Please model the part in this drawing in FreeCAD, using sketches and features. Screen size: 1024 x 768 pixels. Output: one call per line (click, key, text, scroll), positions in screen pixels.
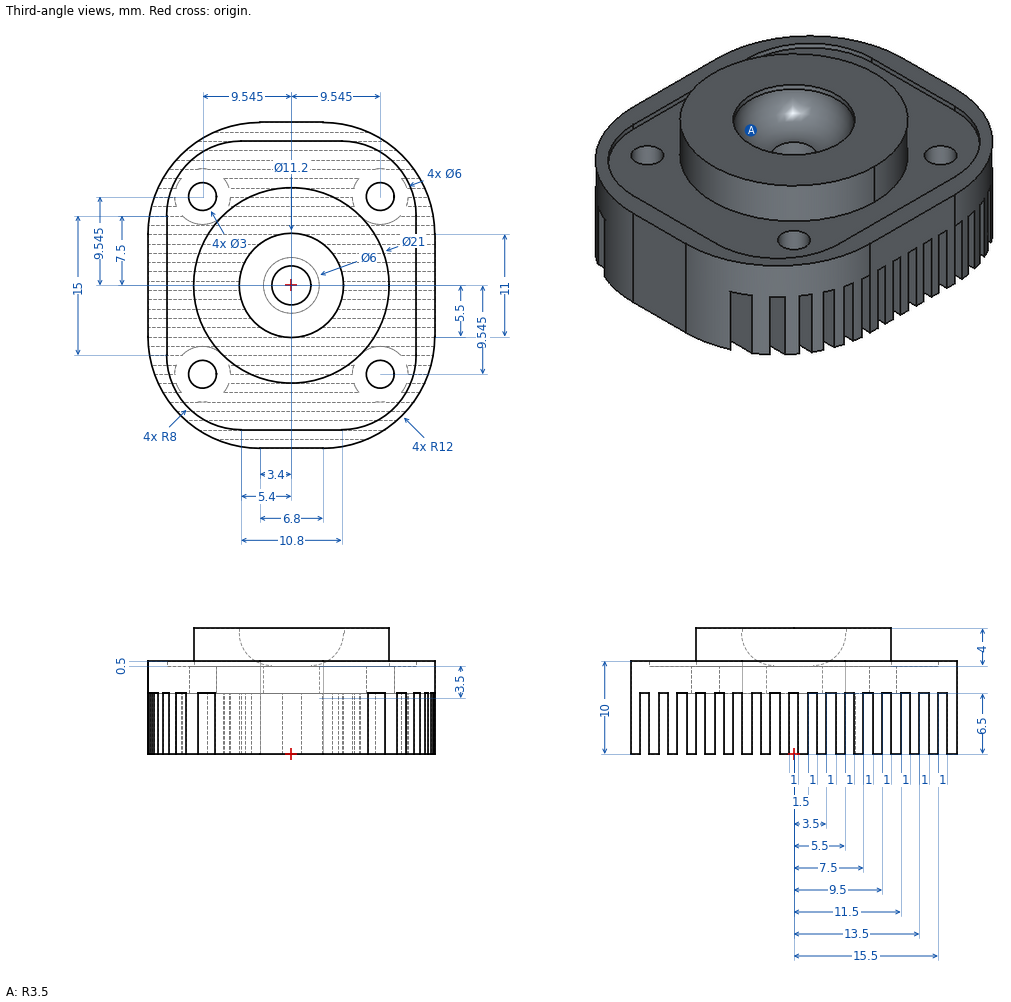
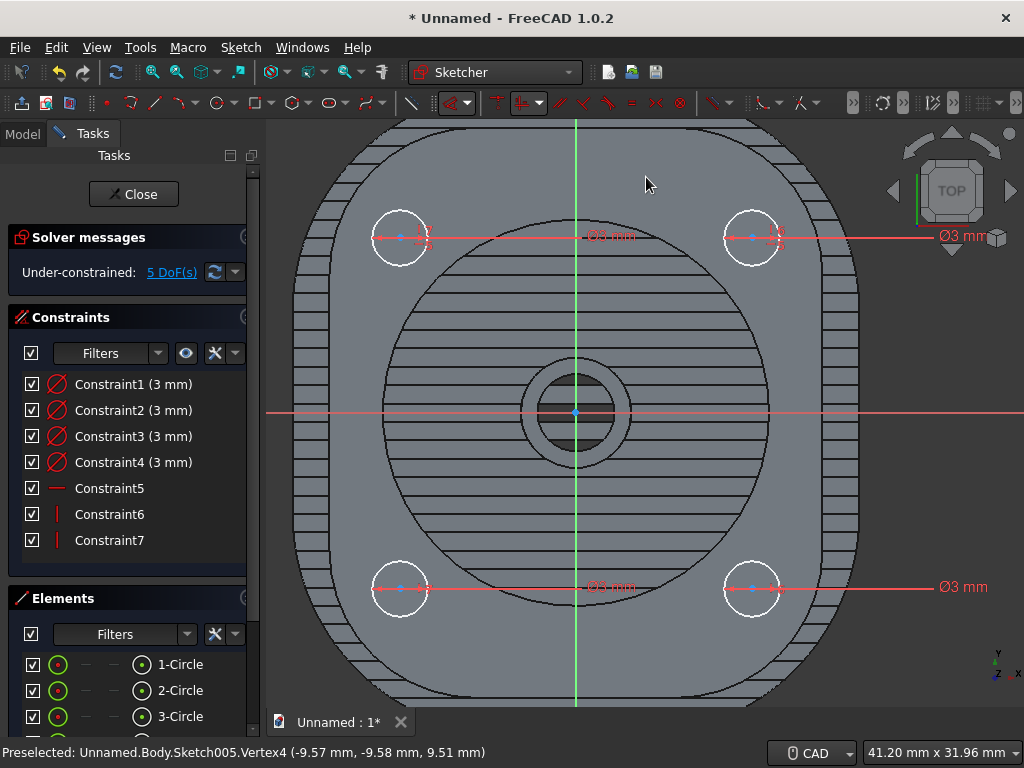
click(752, 589)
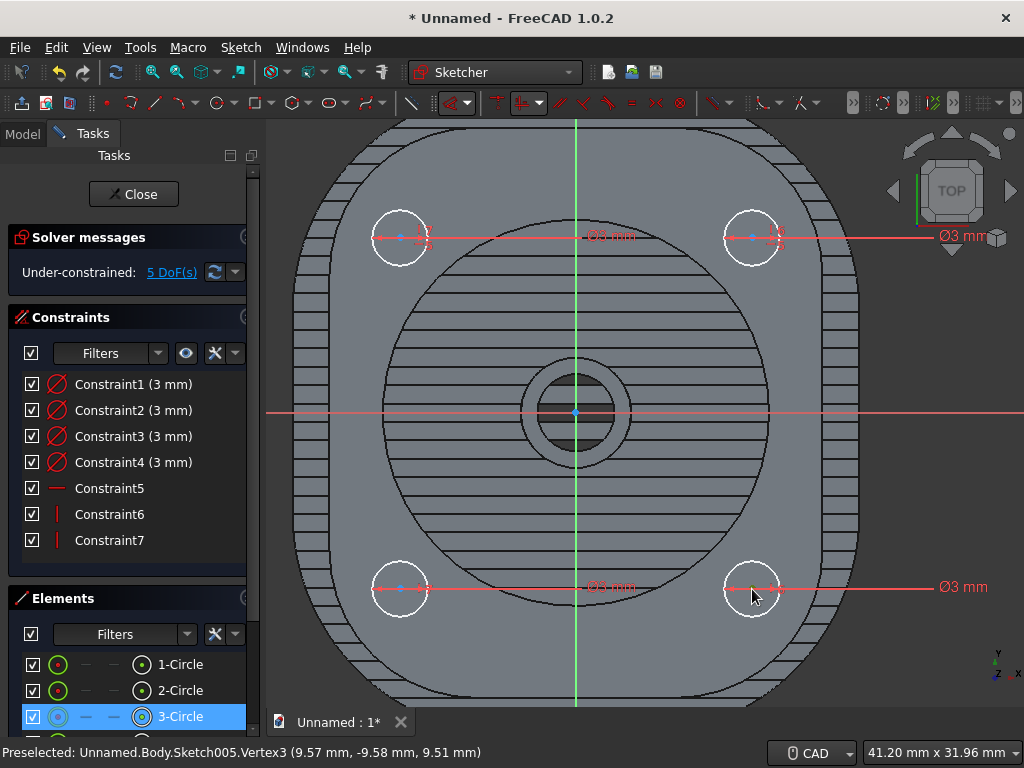
click(400, 589)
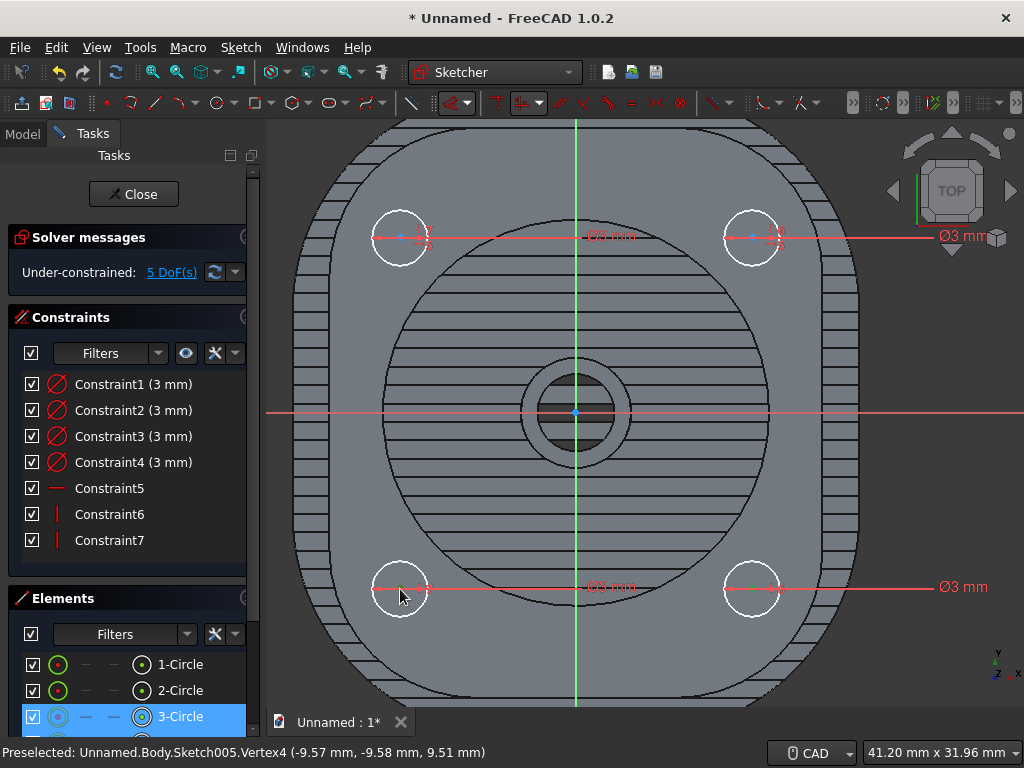
click(542, 104)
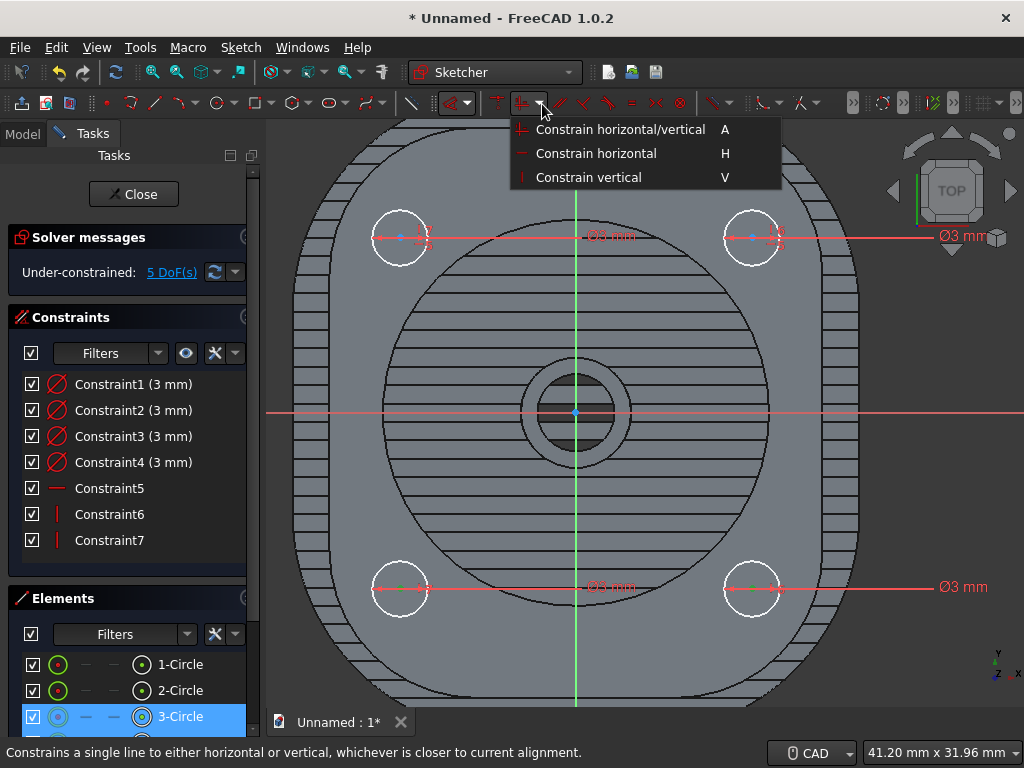
click(646, 153)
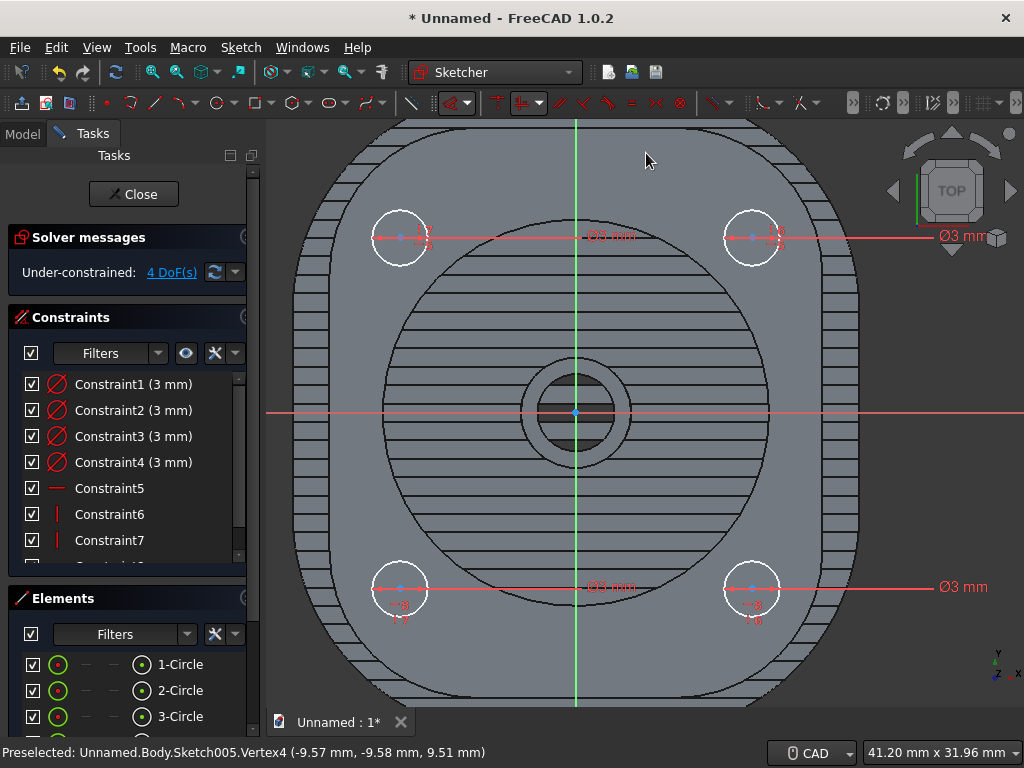
click(400, 238)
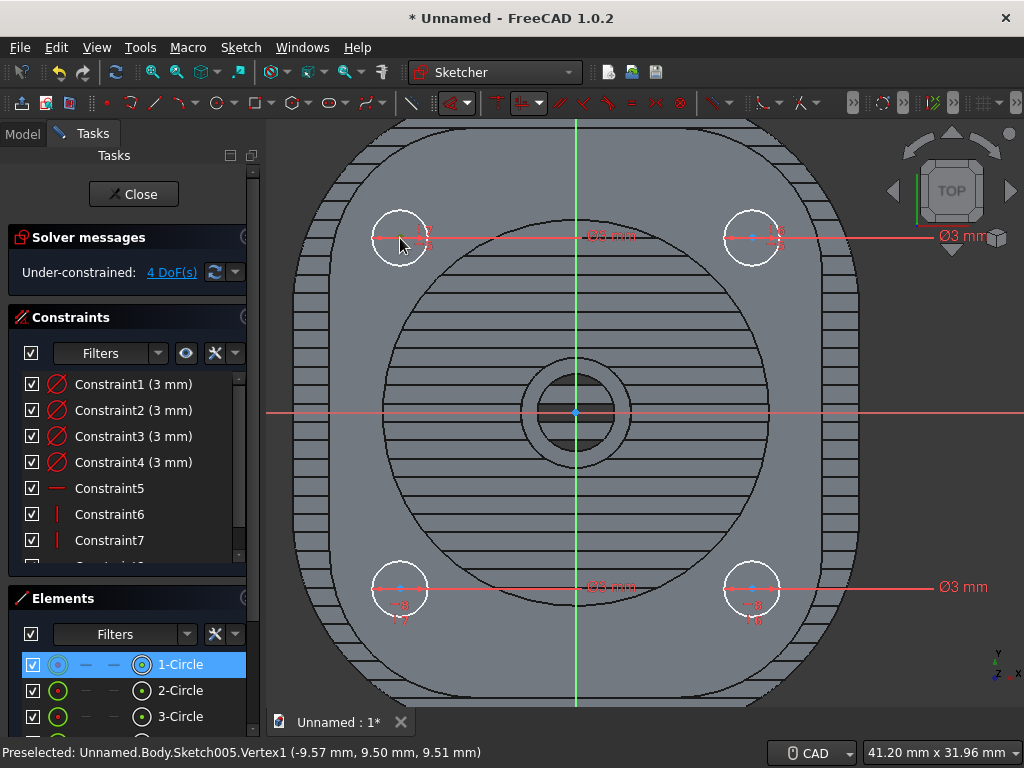
key(l)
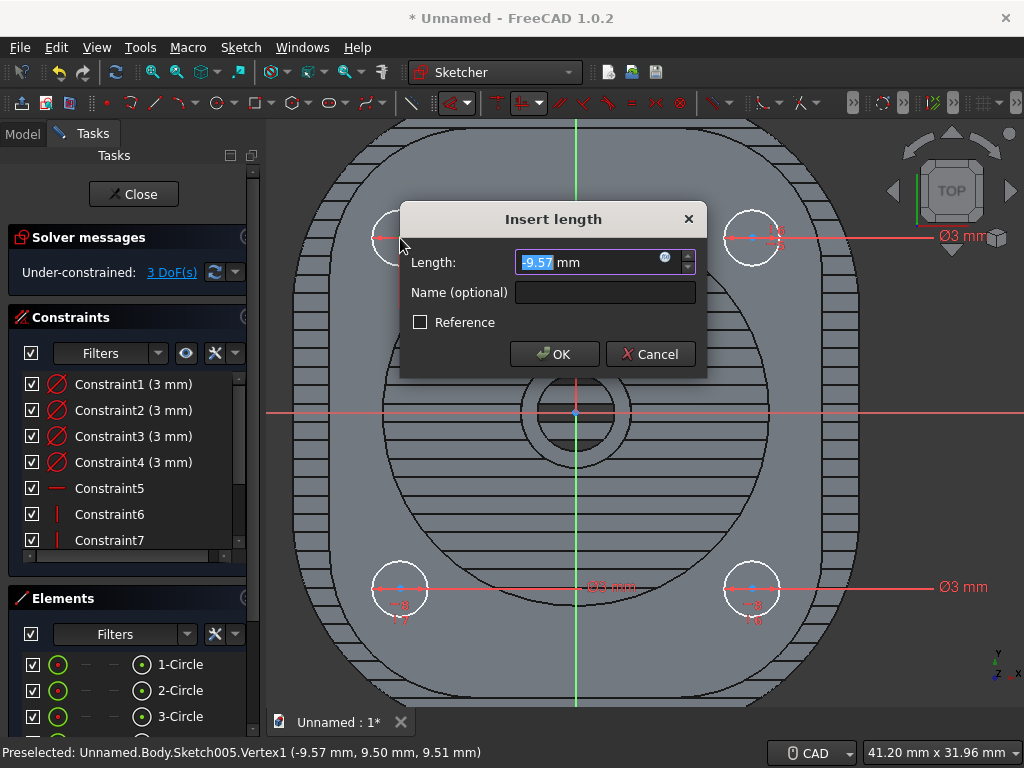
text(-9.545)
key(Return)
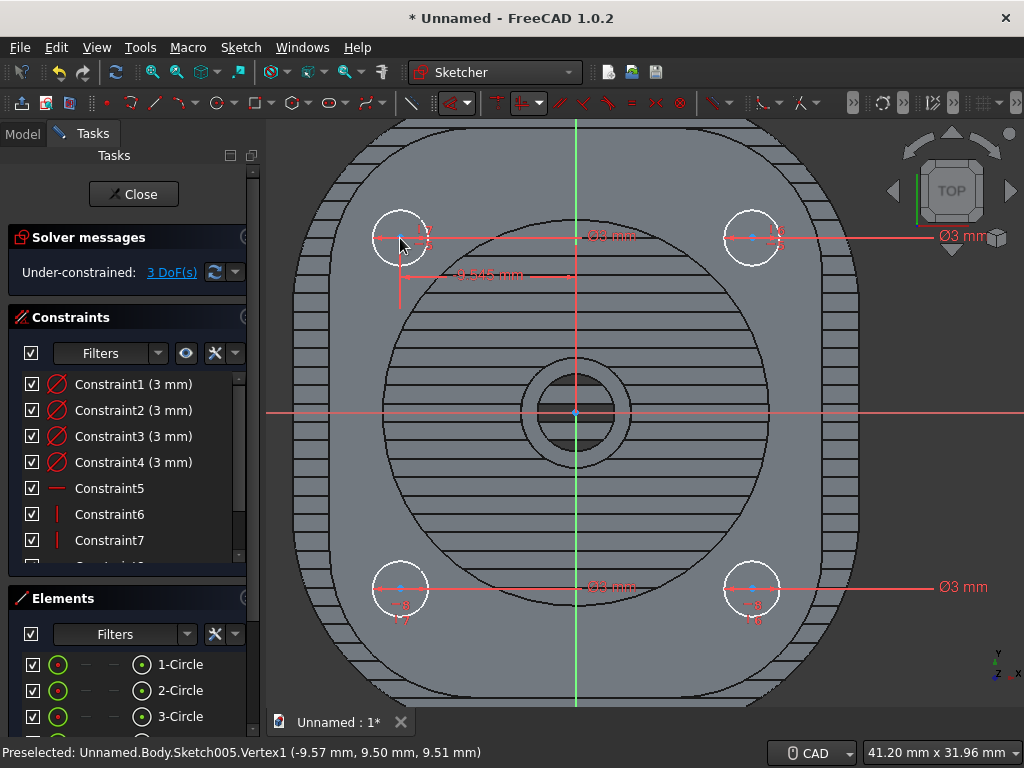
click(400, 238)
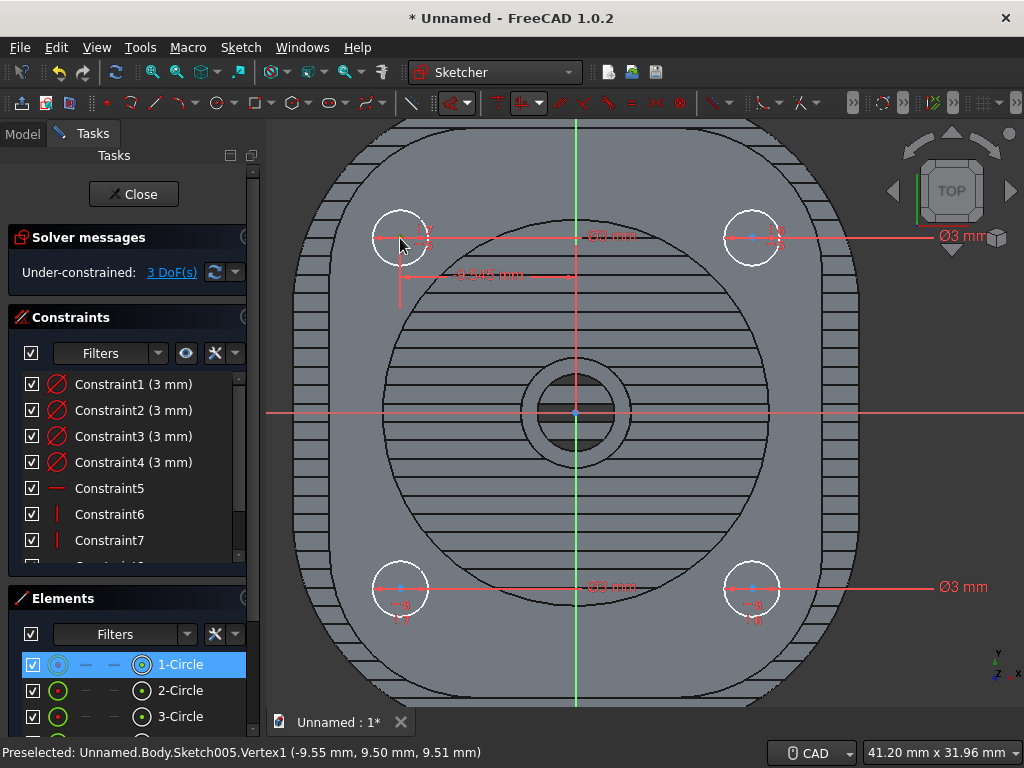
key(i)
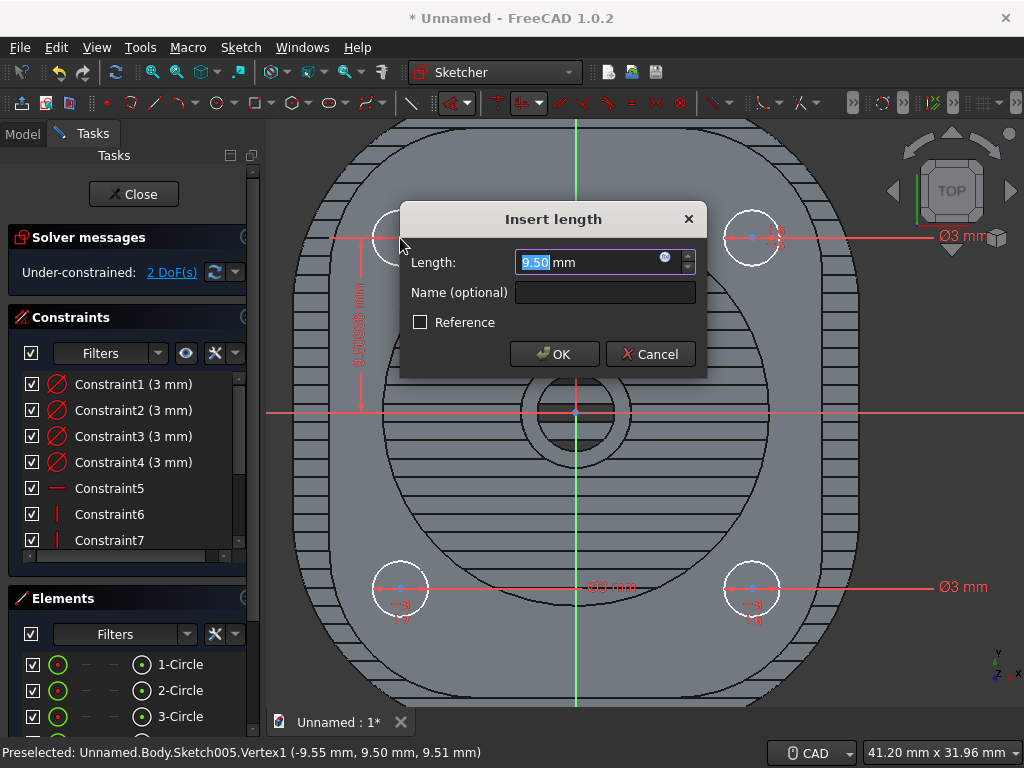
text(9.545)
key(Return)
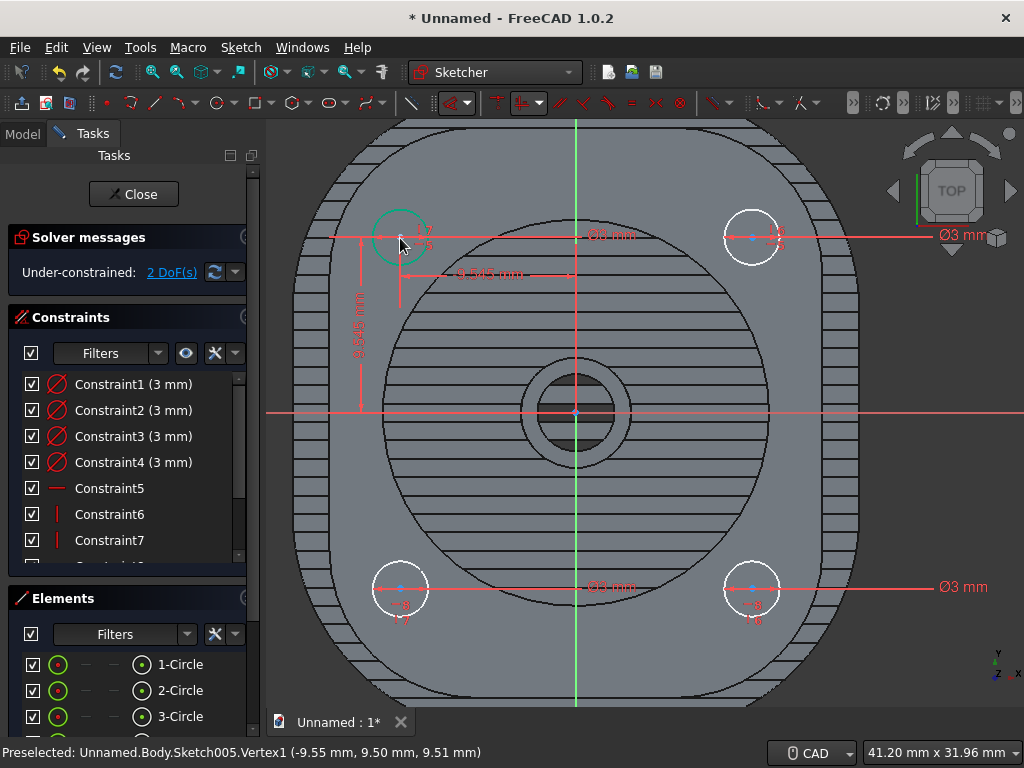
click(752, 237)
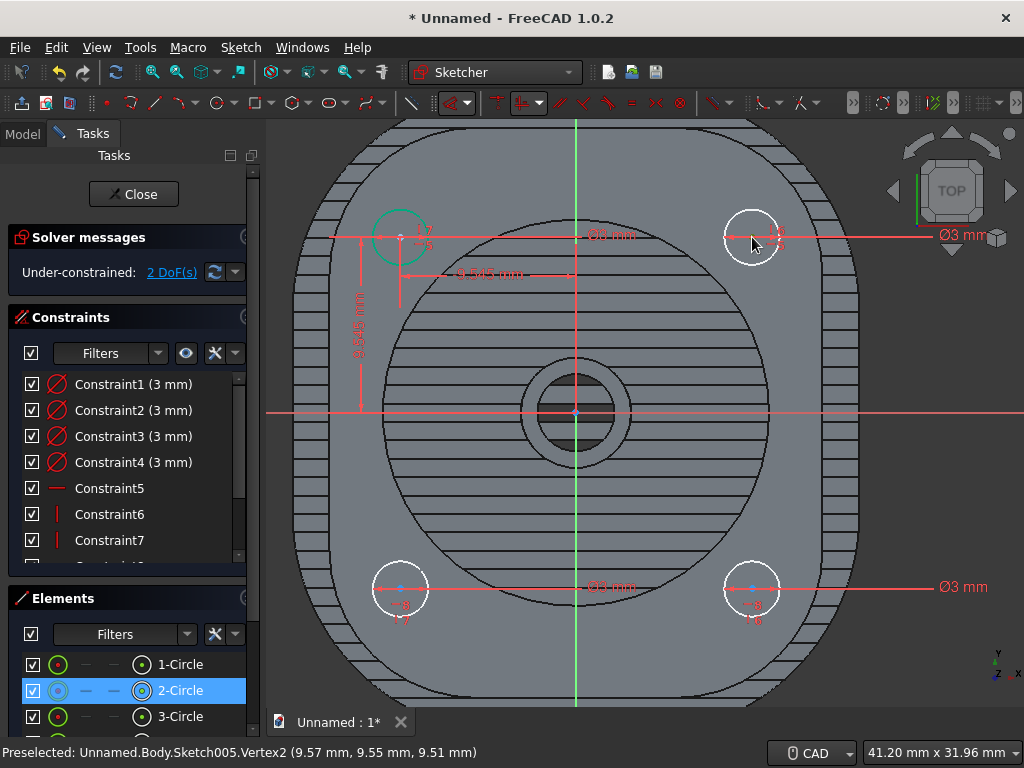
click(470, 104)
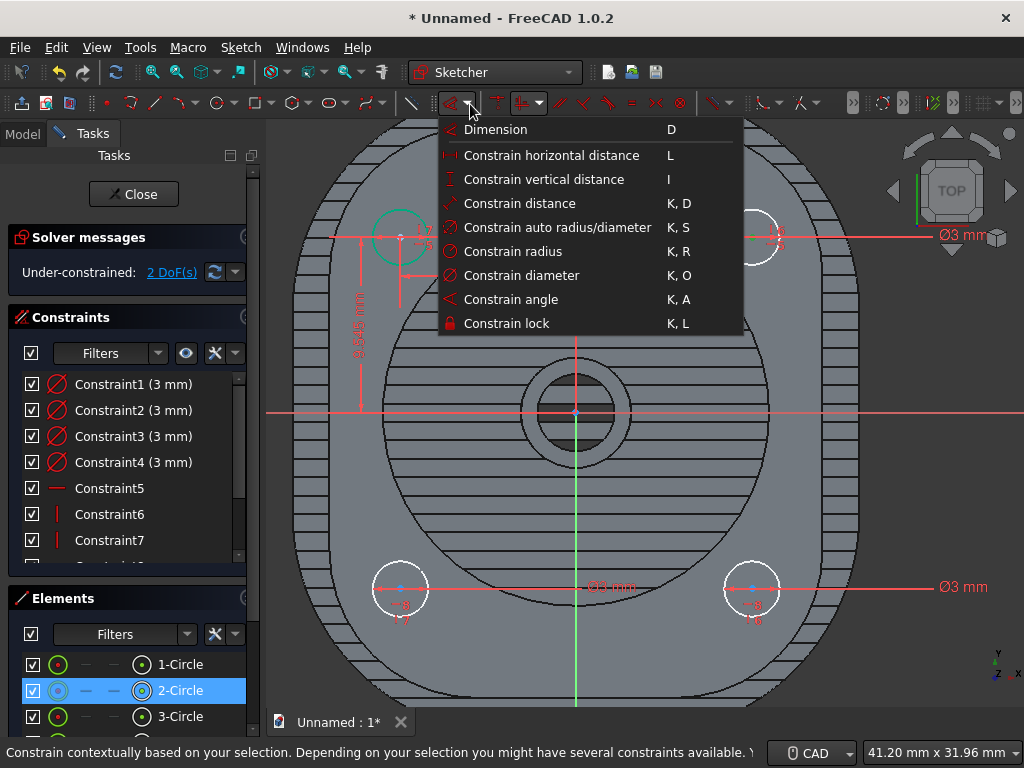
click(591, 155)